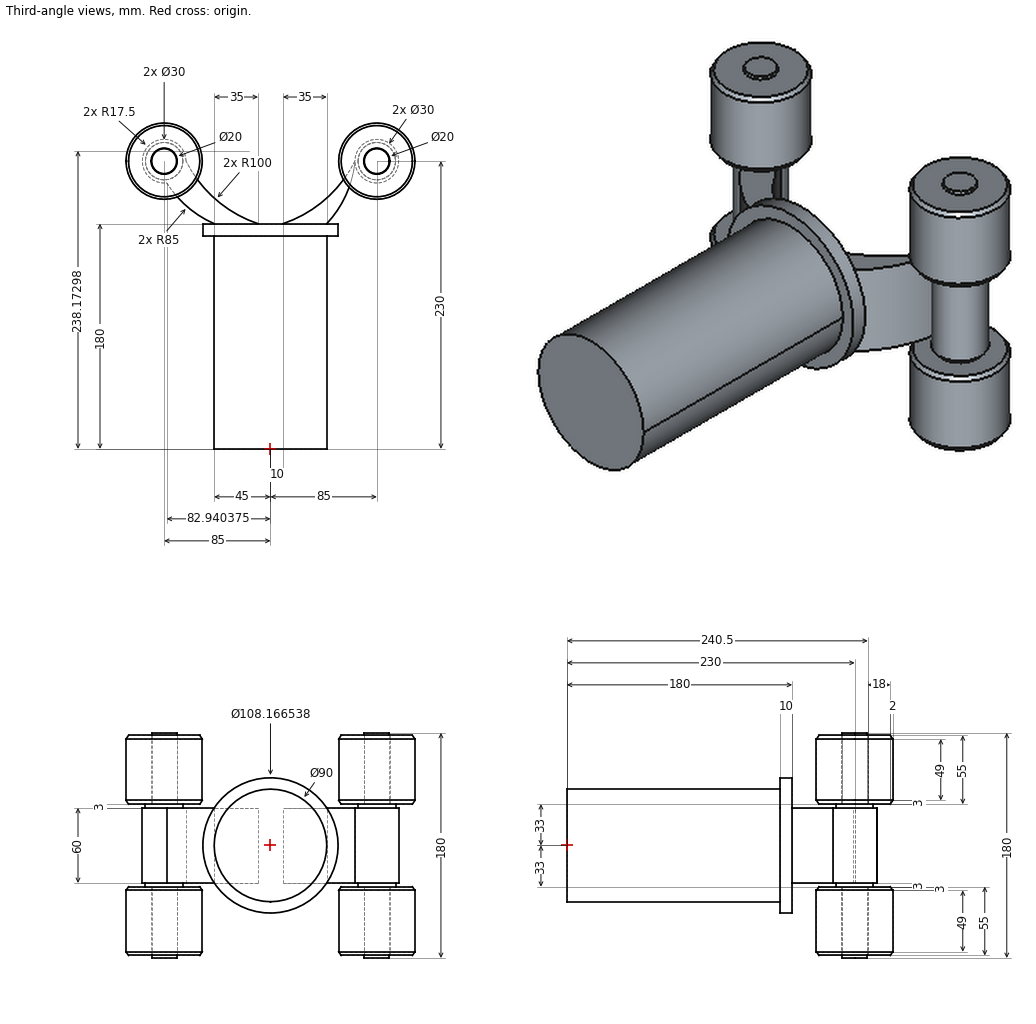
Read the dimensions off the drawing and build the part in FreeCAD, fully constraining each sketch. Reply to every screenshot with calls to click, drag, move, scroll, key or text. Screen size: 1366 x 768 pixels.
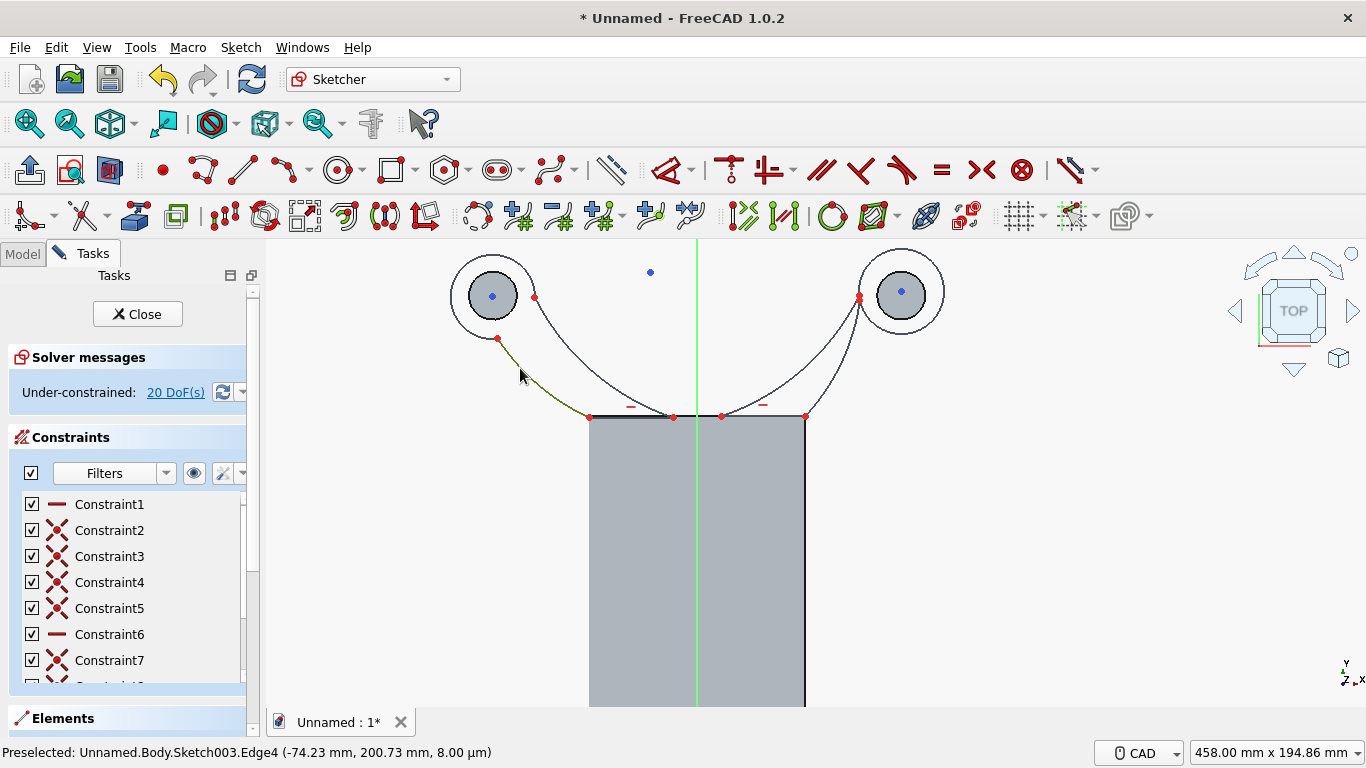
click(829, 385)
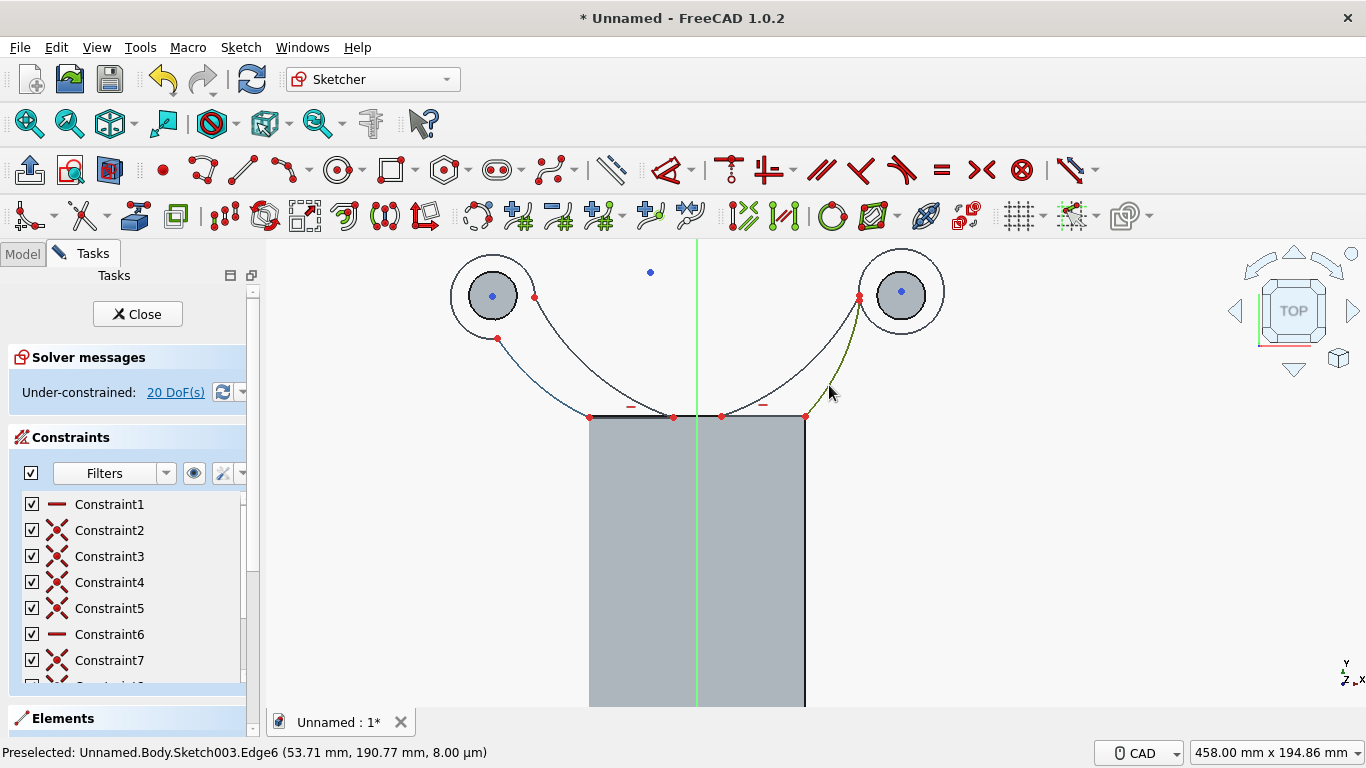
click(942, 170)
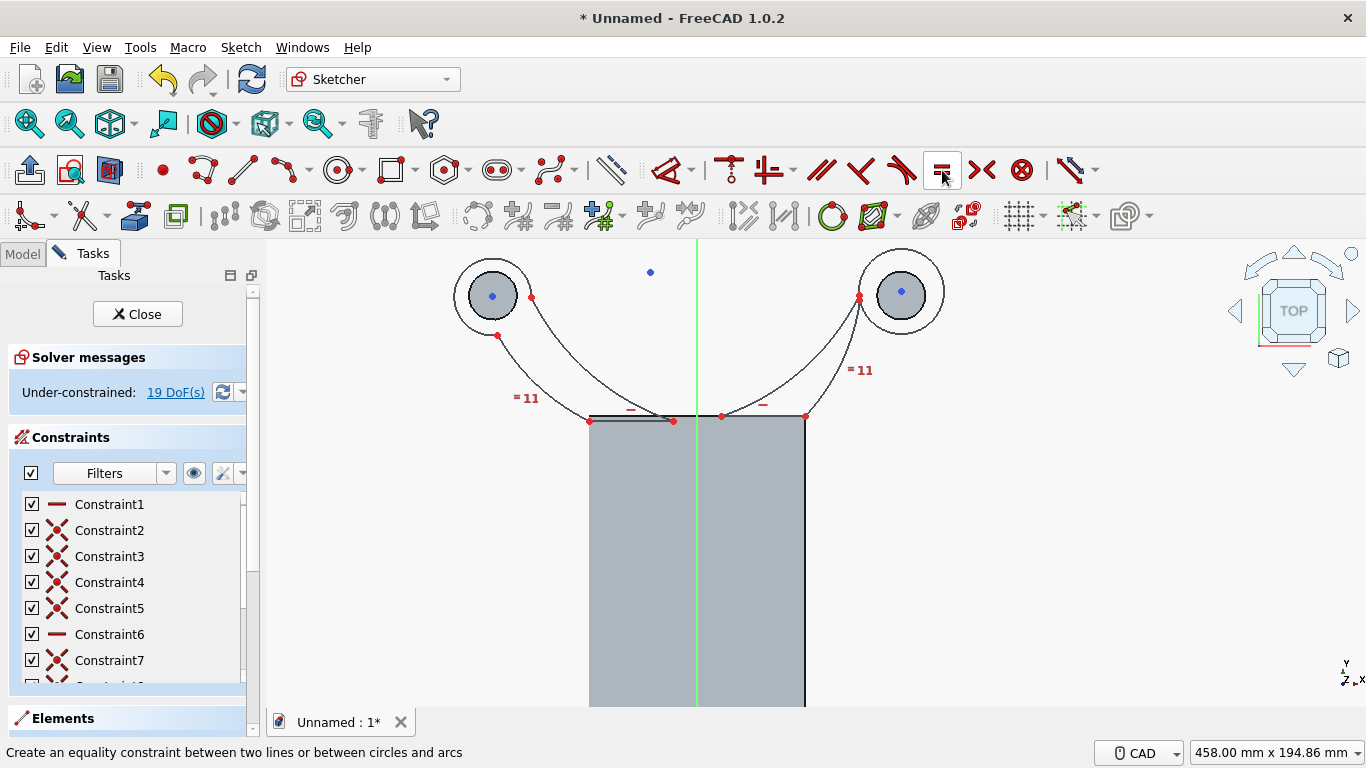
click(455, 306)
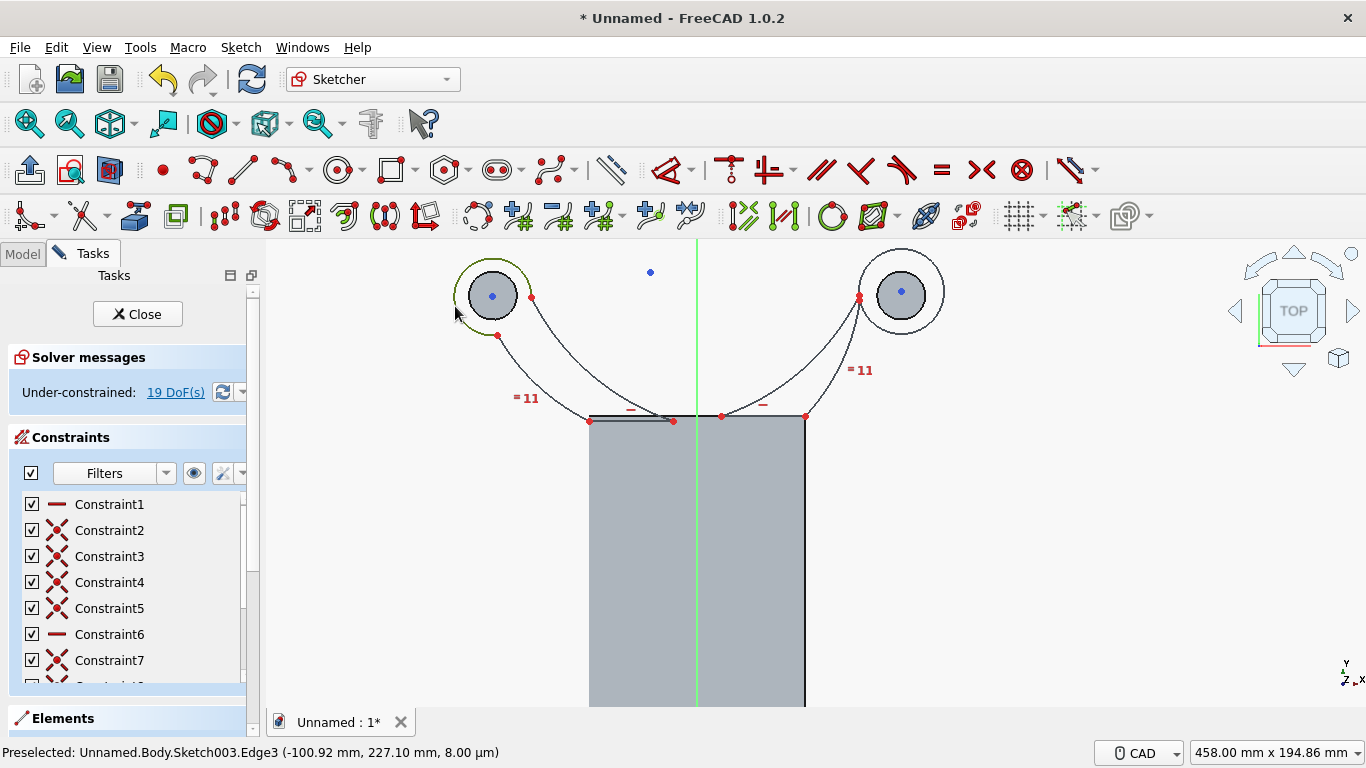
click(922, 329)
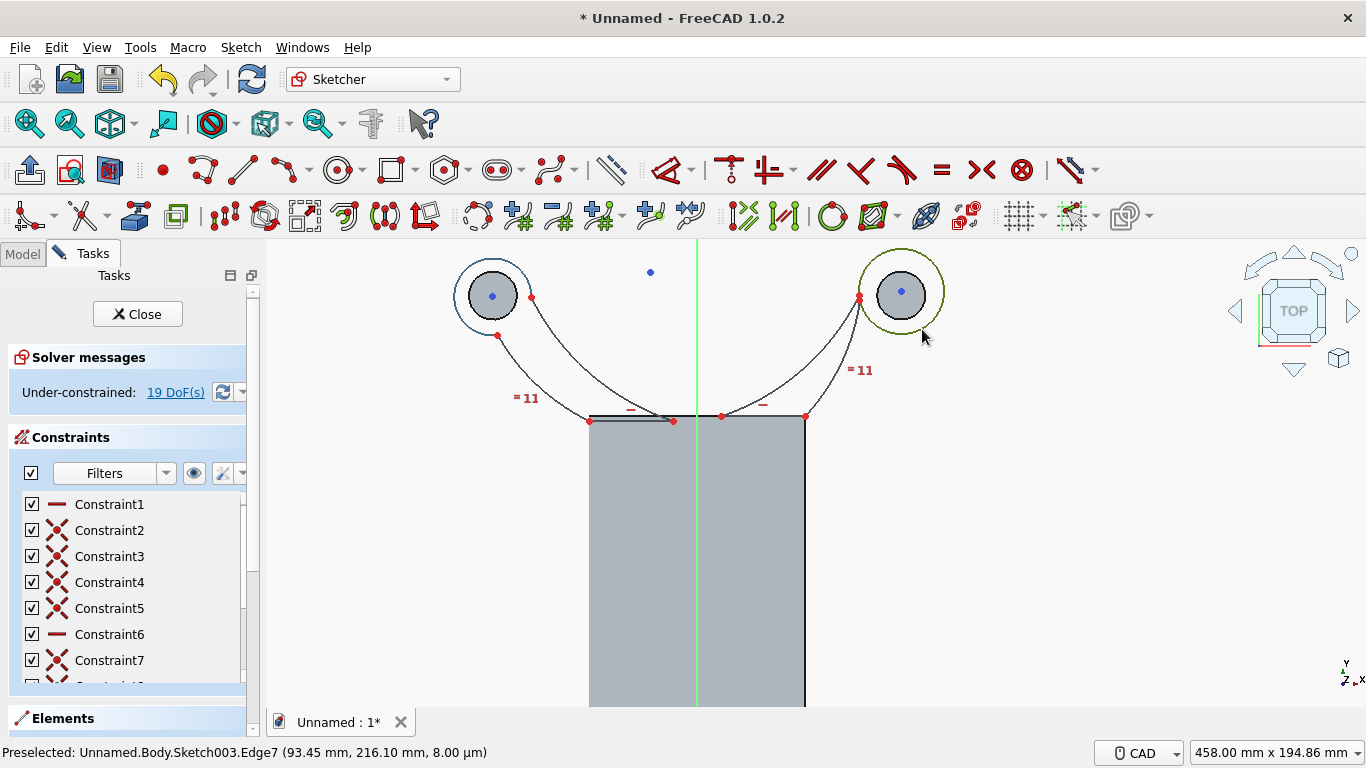
click(942, 170)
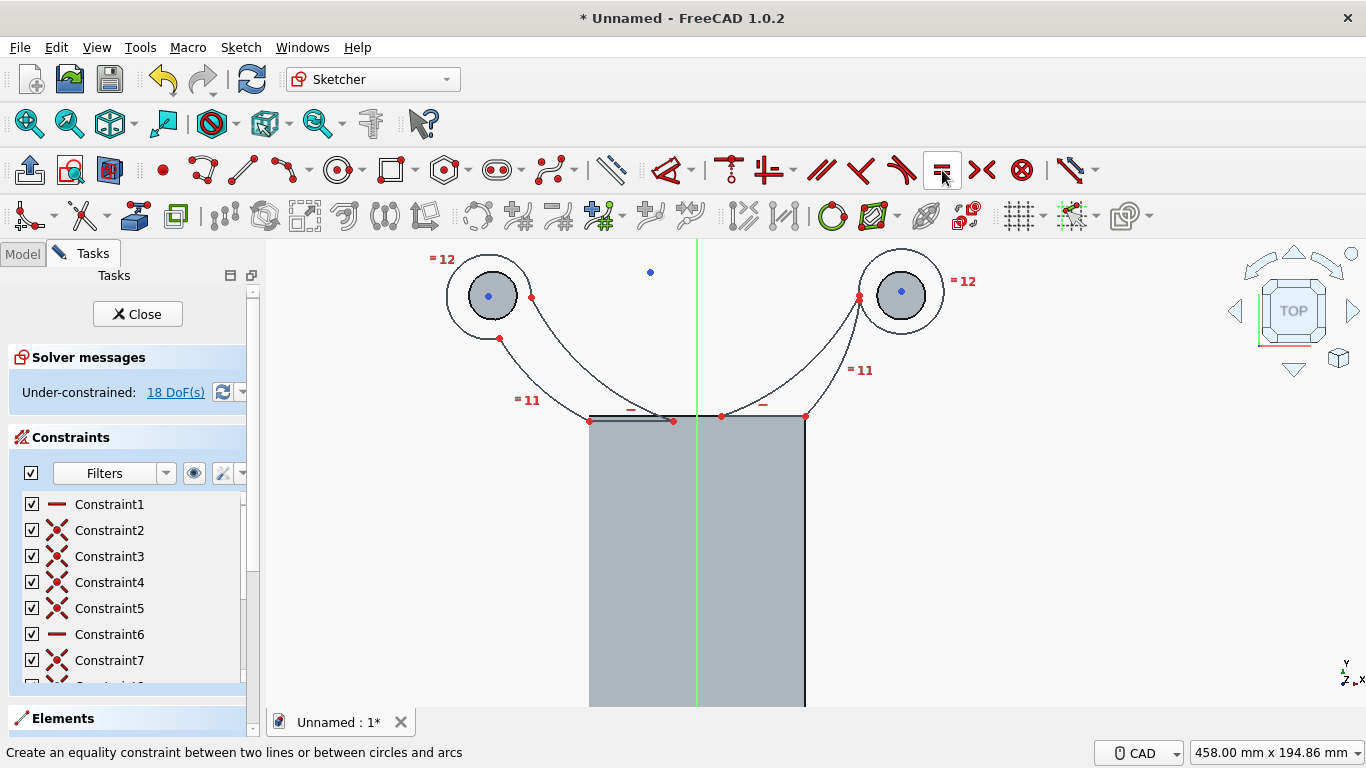
click(563, 346)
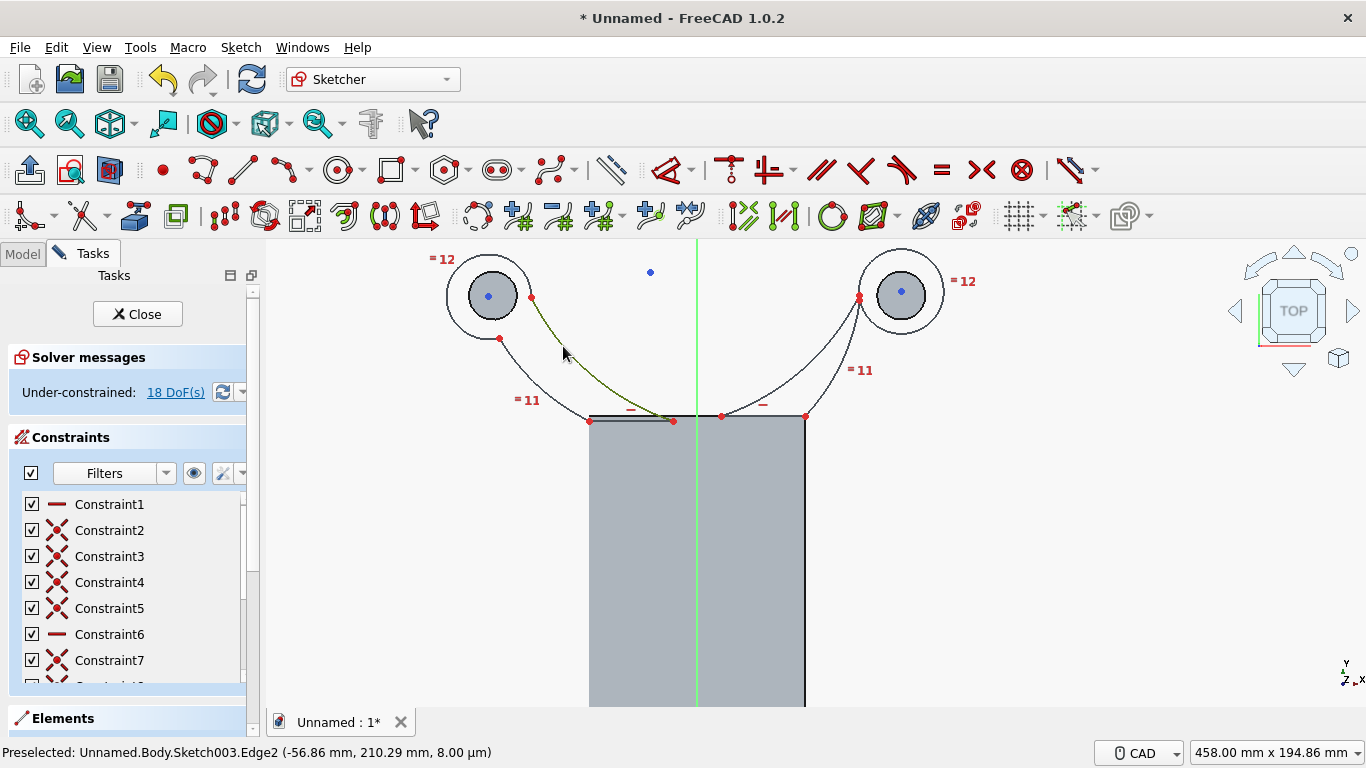
click(772, 392)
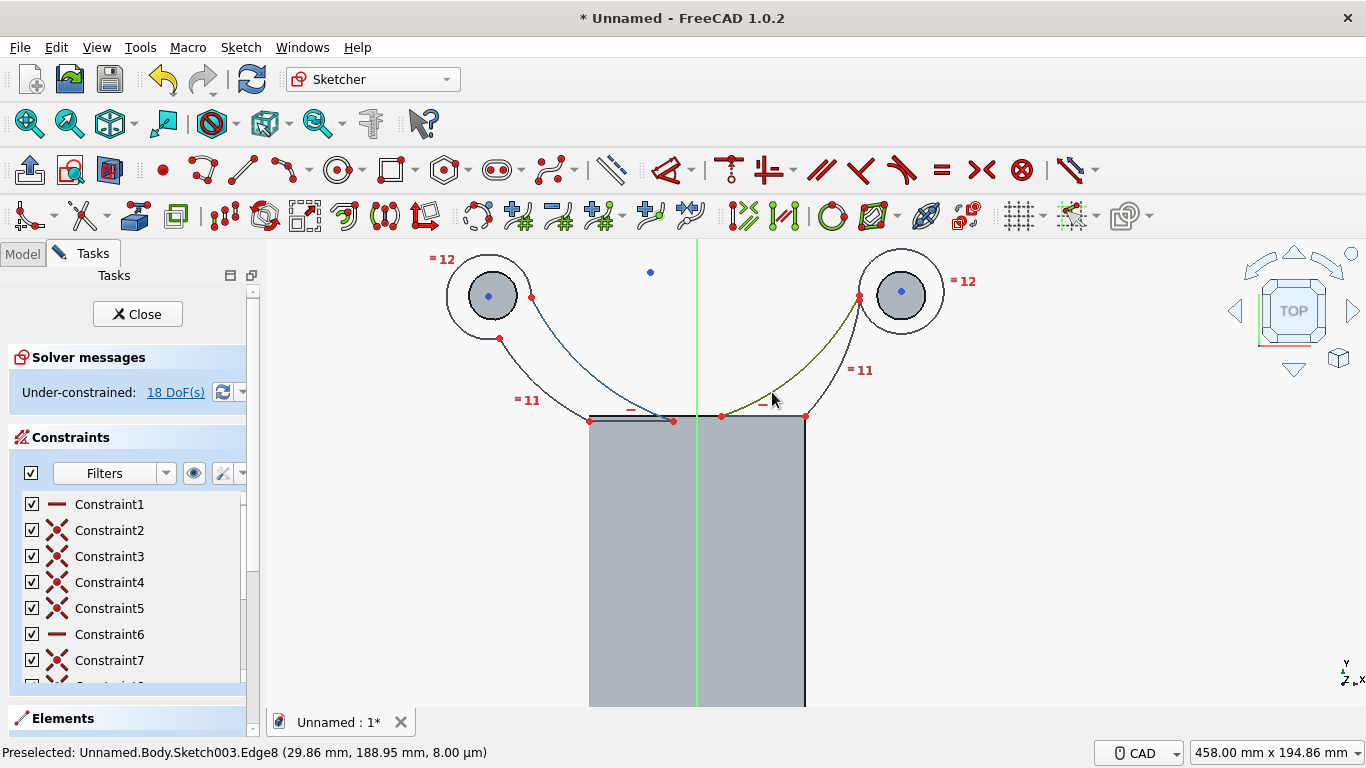
click(942, 170)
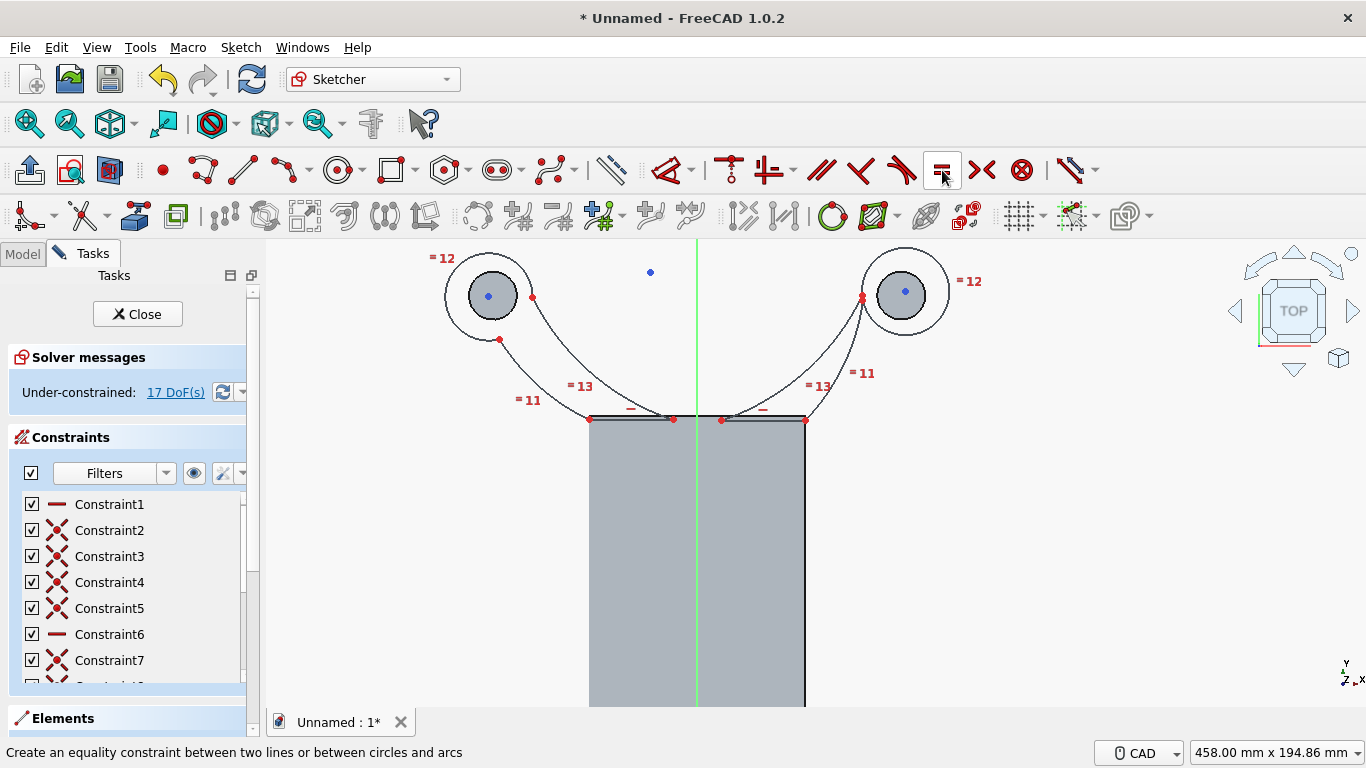
click(666, 170)